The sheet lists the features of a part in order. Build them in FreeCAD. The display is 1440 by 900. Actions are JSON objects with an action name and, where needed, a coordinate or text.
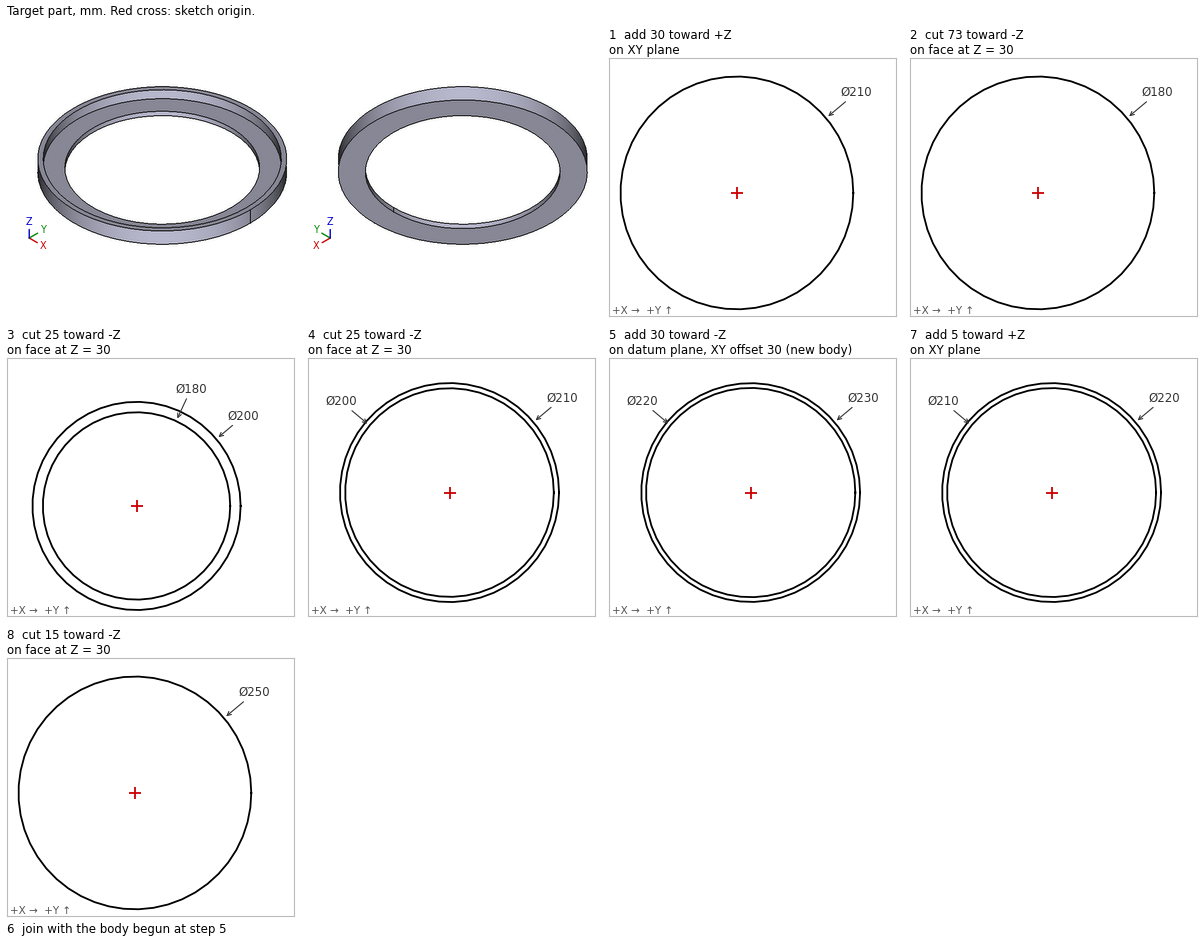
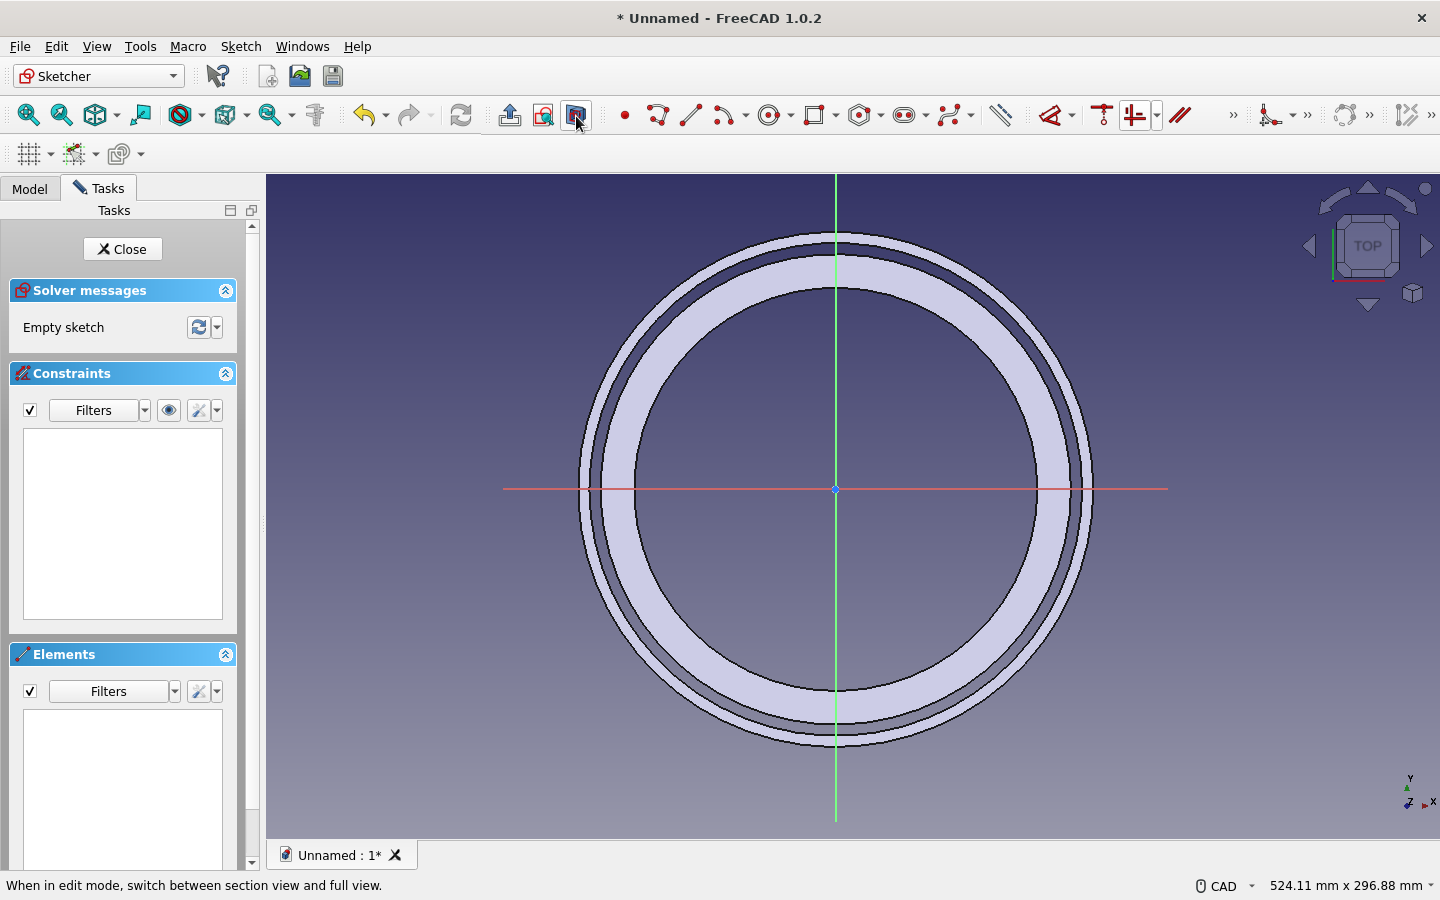
{"action": "left_click", "coordinate": [768, 116]}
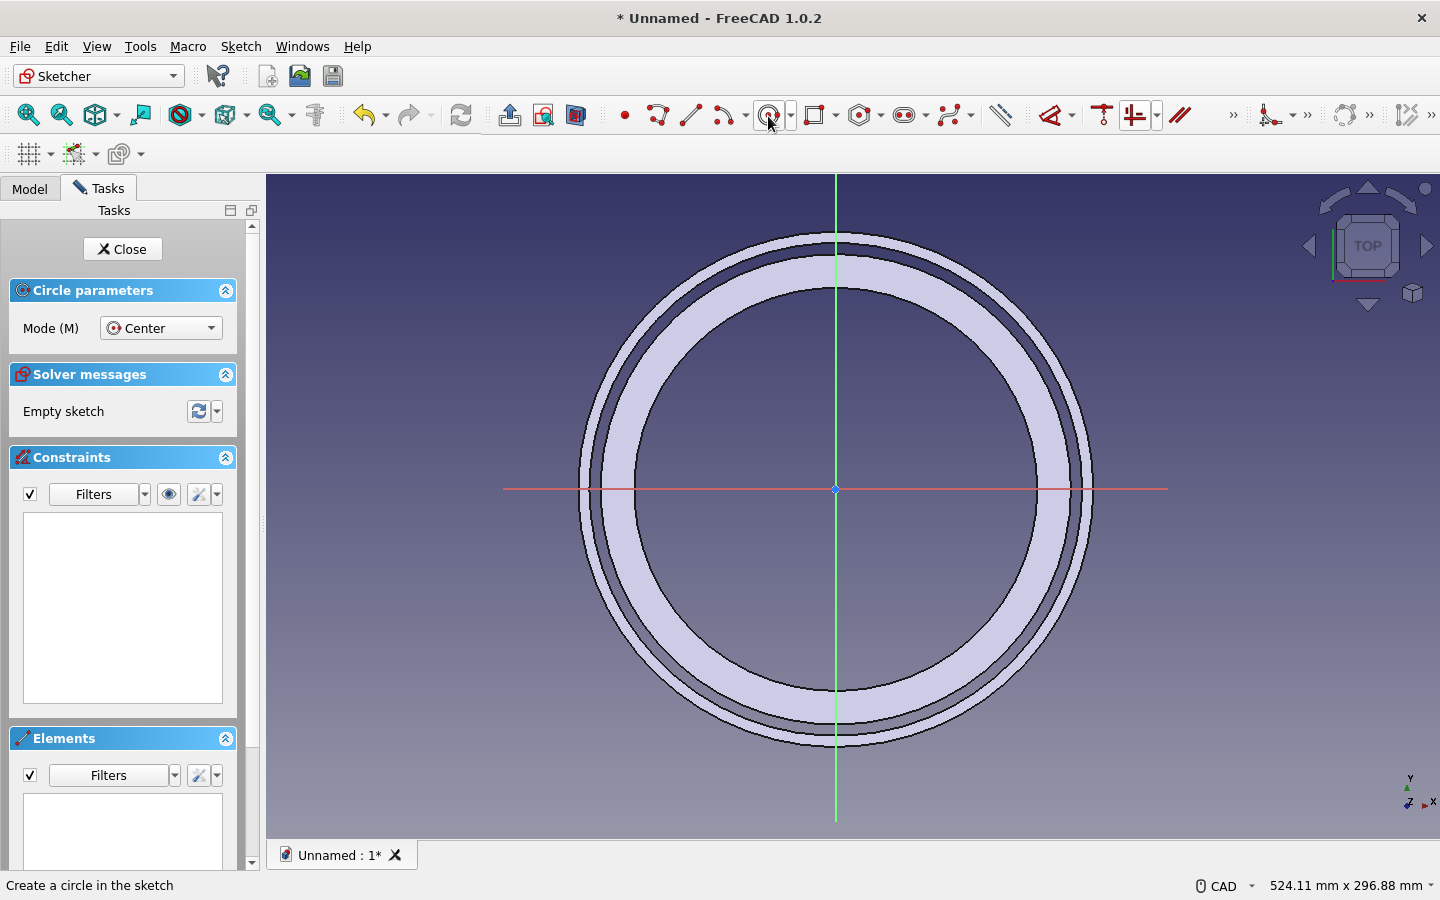
{"action": "left_click", "coordinate": [836, 489]}
{"action": "mouse_move", "coordinate": [1010, 315]}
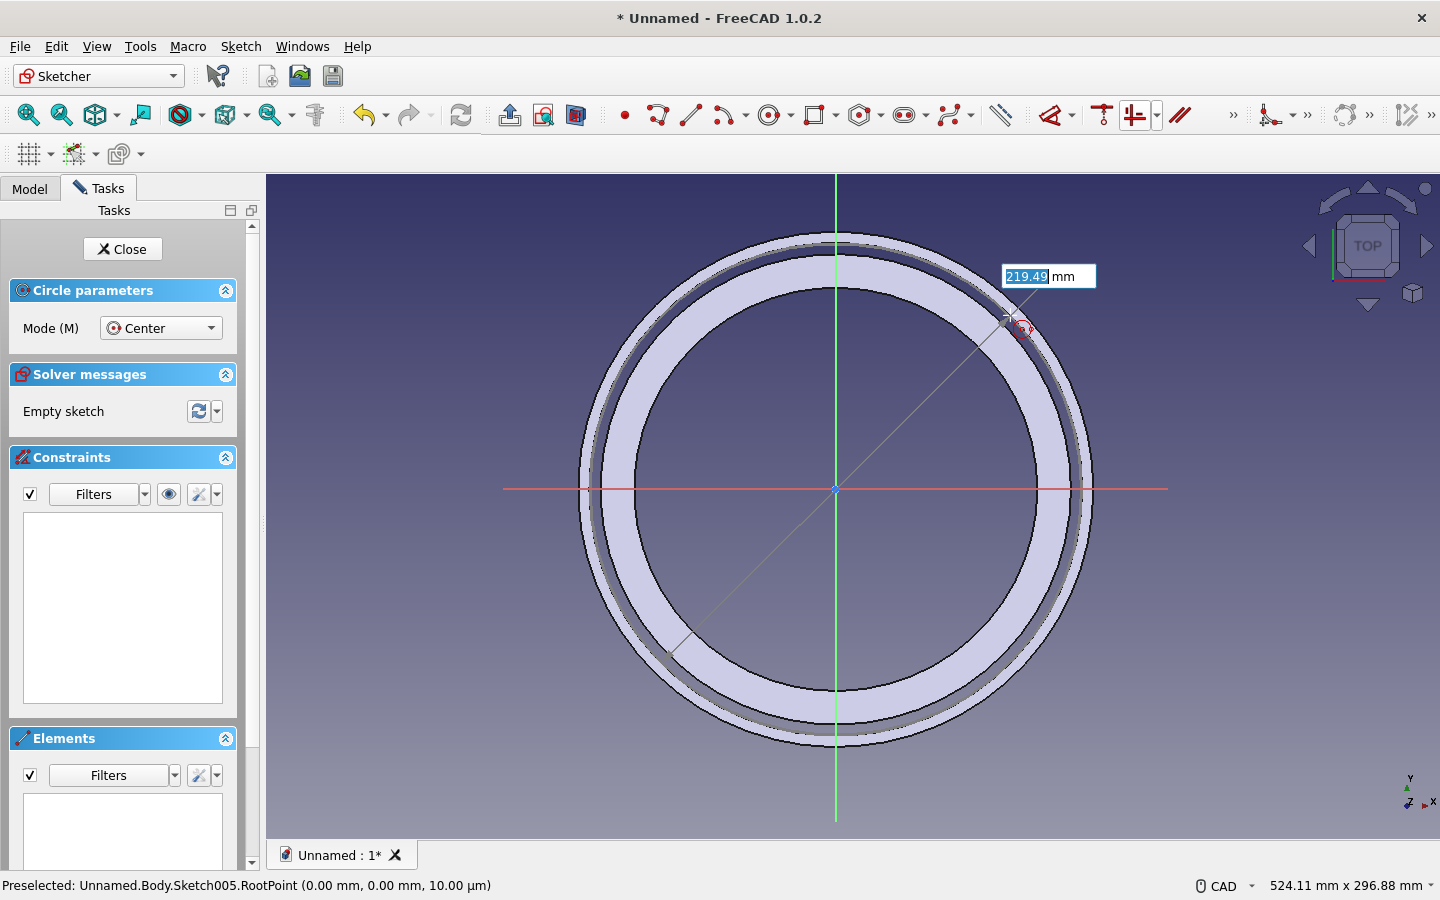
{"action": "type", "text": "220"}
{"action": "key", "text": "Return"}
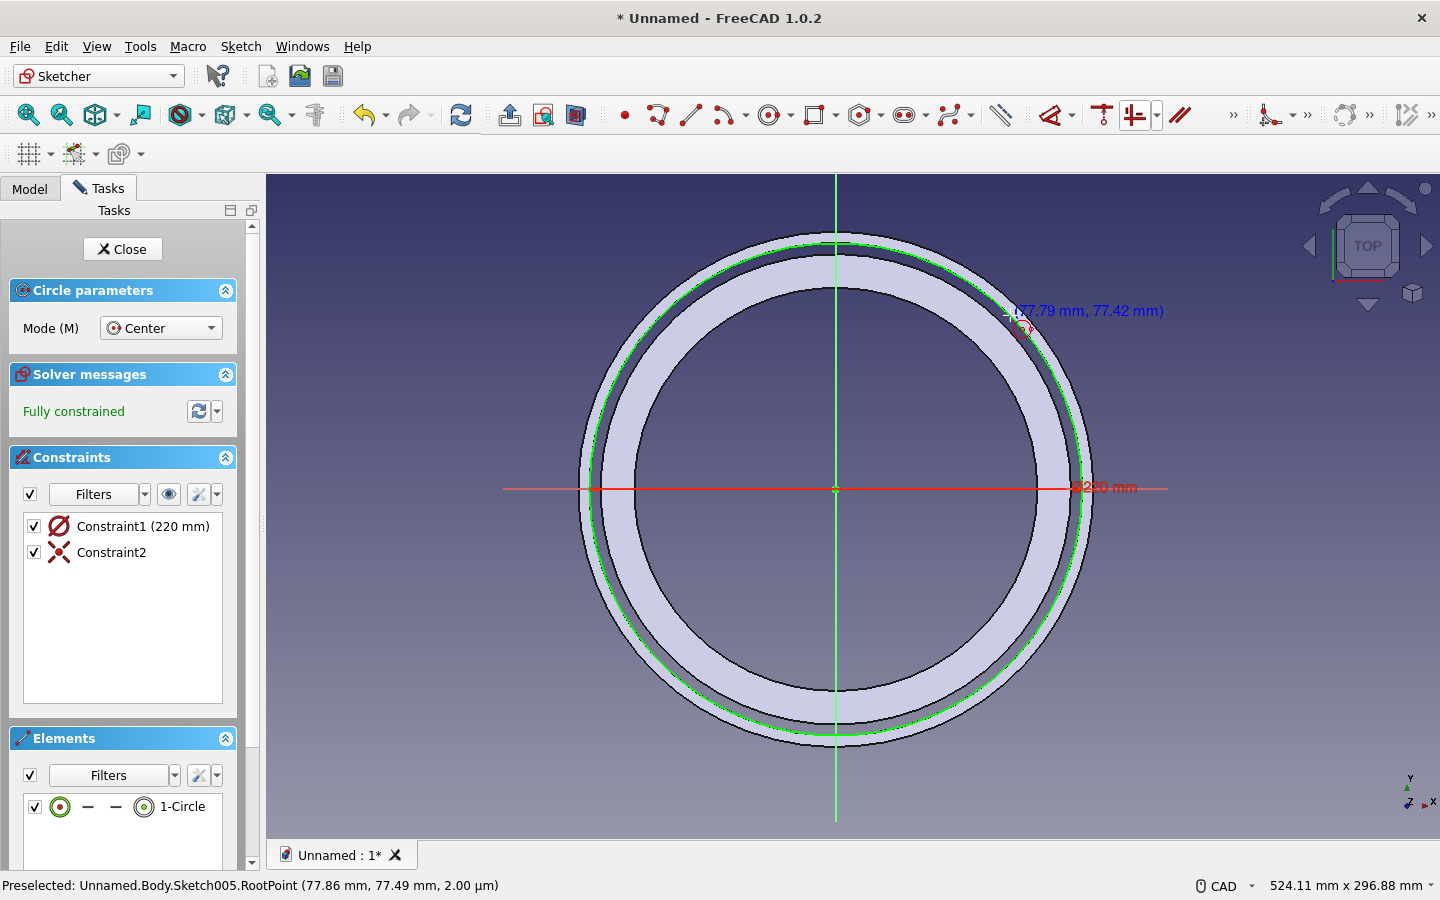
{"action": "left_click", "coordinate": [836, 489]}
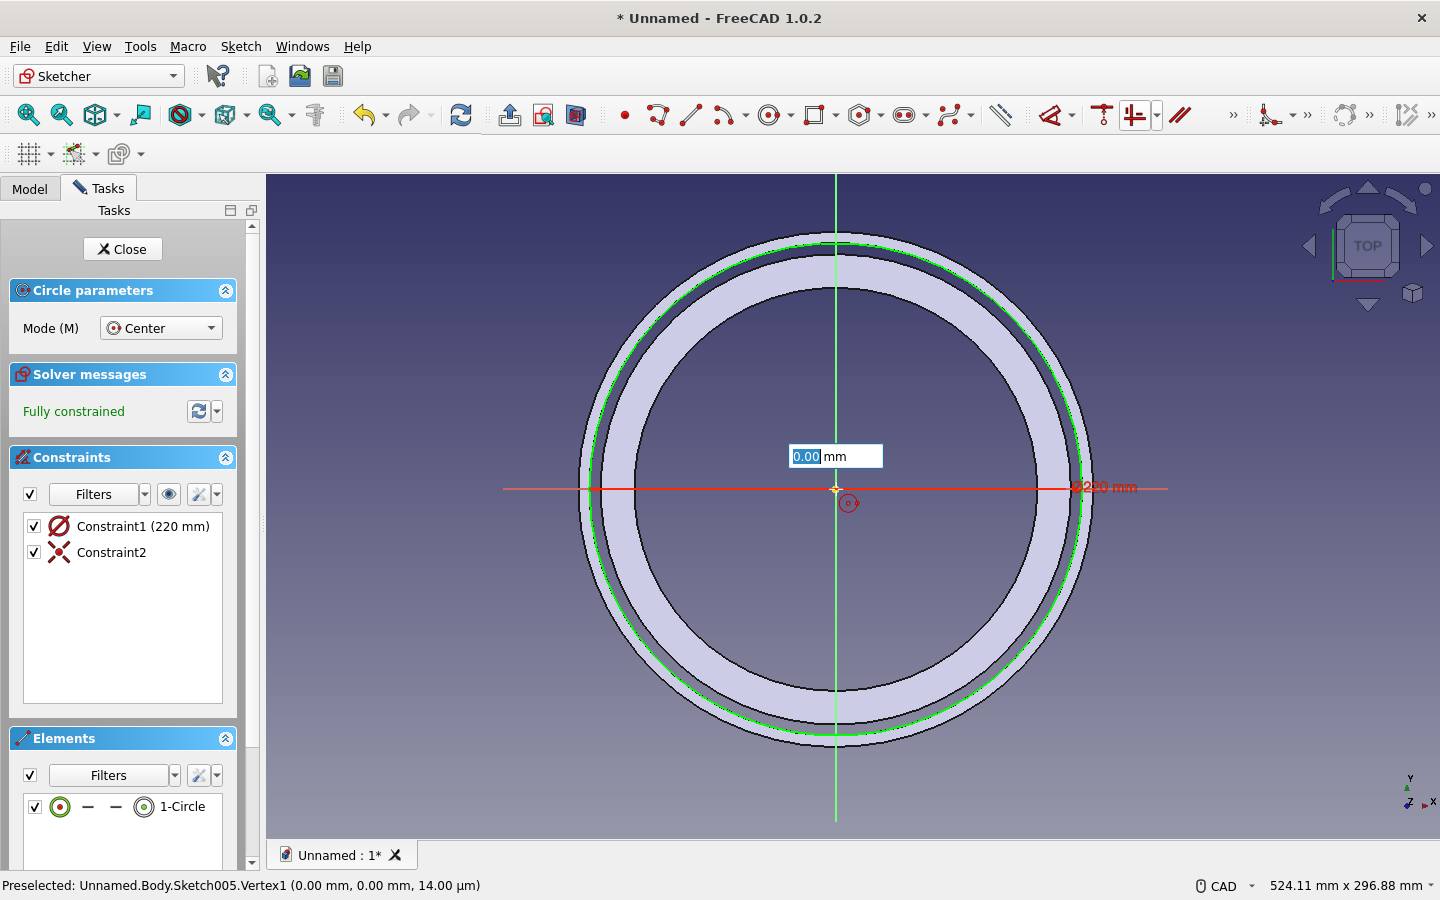
{"action": "scroll", "coordinate": [1002, 323], "scroll_direction": "up", "scroll_amount": 2}
{"action": "mouse_move", "coordinate": [1002, 323]}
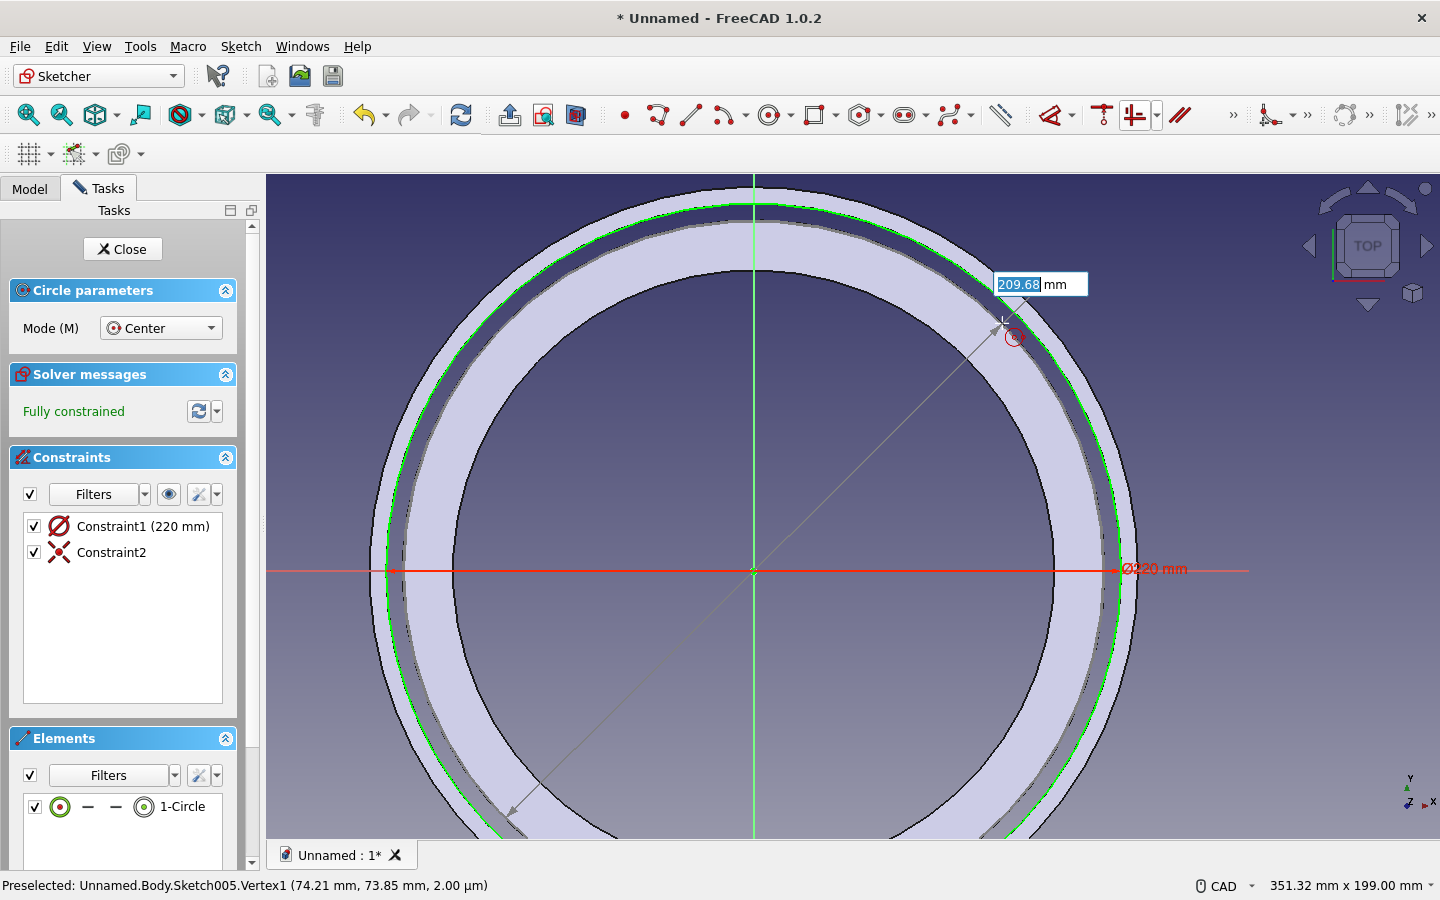
{"action": "type", "text": "210"}
{"action": "key", "text": "Return"}
{"action": "key", "text": "Escape"}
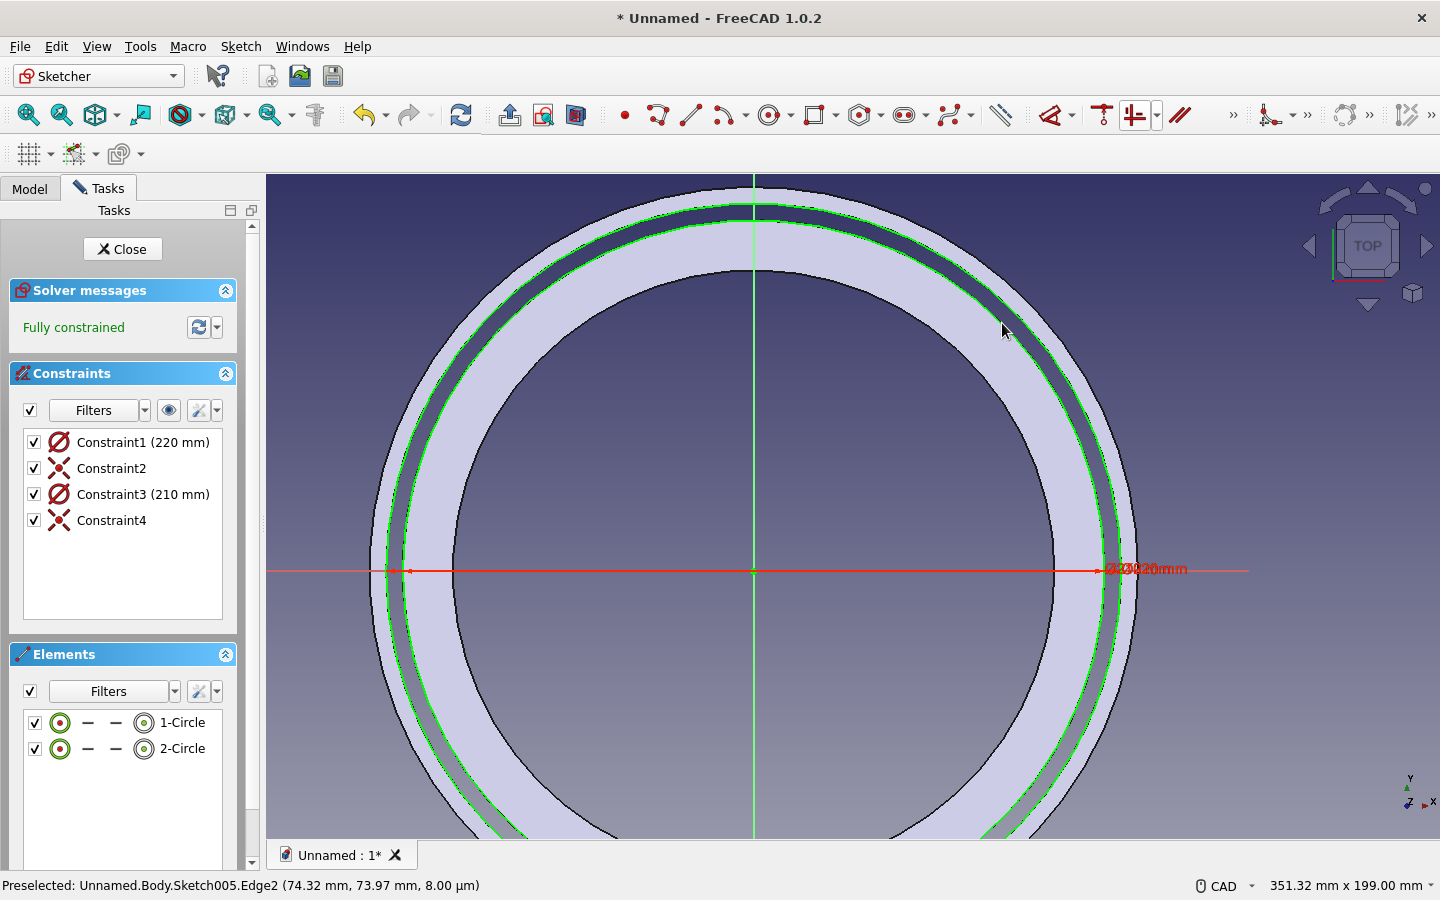
{"action": "left_click", "coordinate": [123, 249]}